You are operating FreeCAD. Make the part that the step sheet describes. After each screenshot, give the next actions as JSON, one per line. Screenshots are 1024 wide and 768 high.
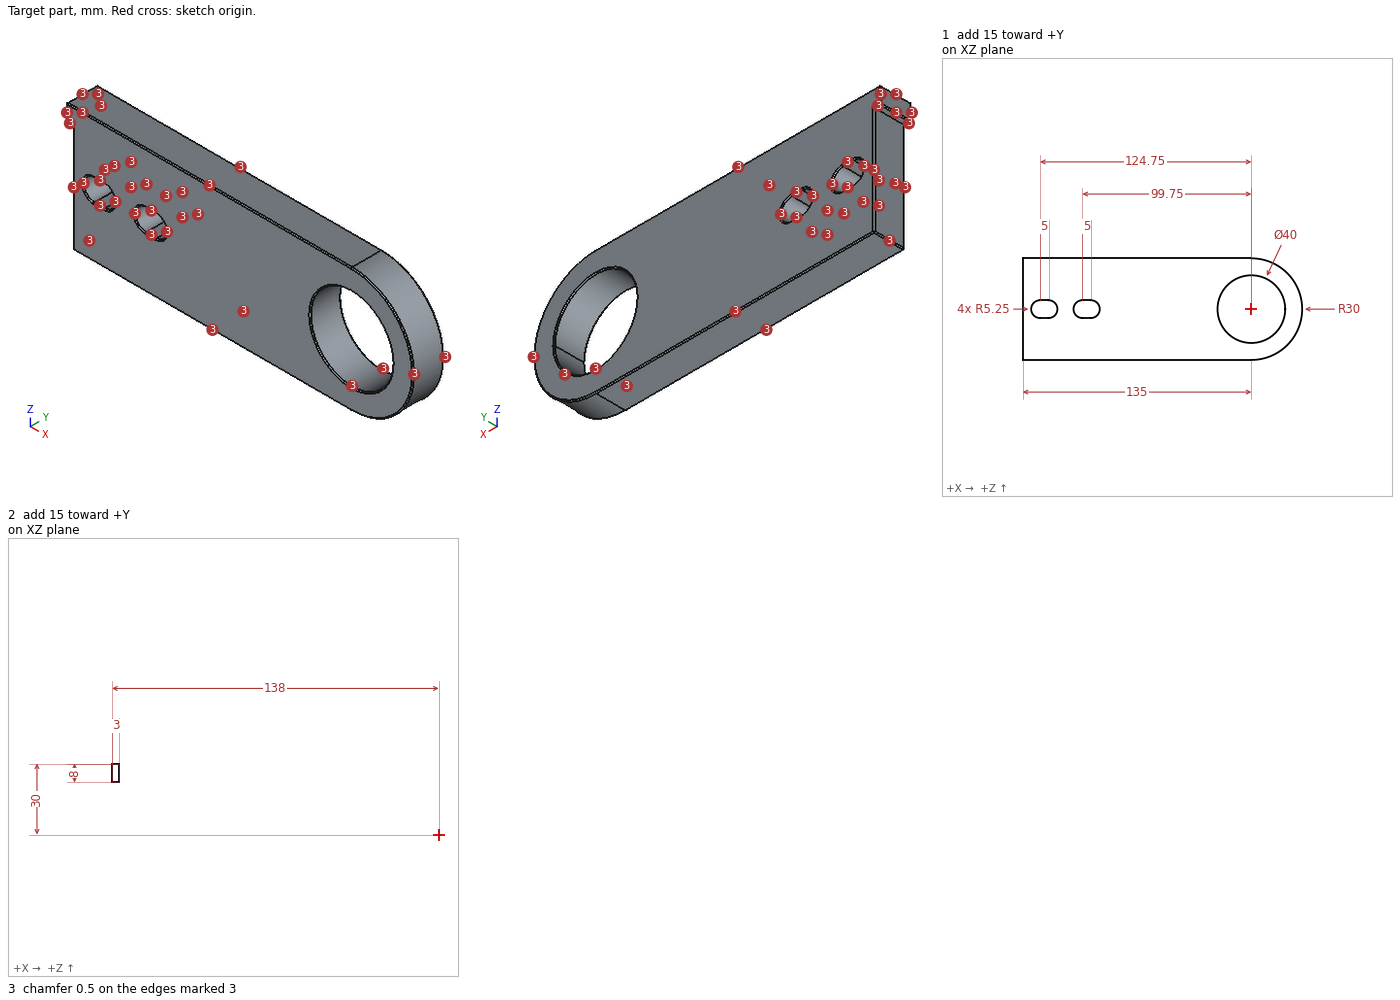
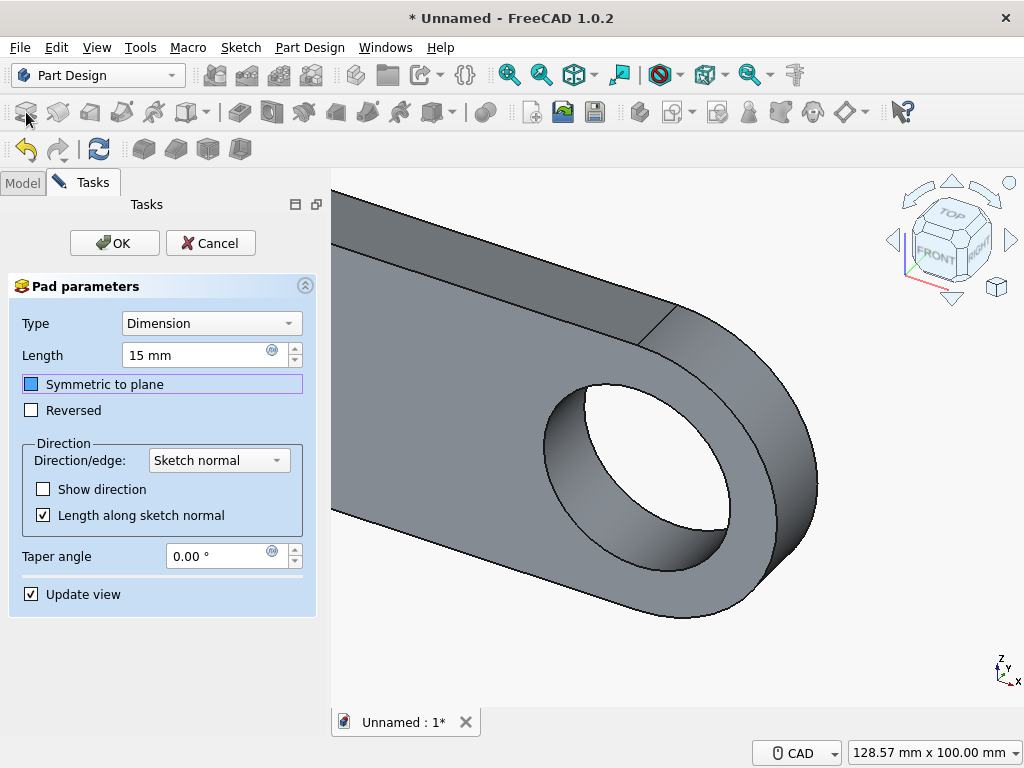
{"action": "left_click", "coordinate": [30, 410]}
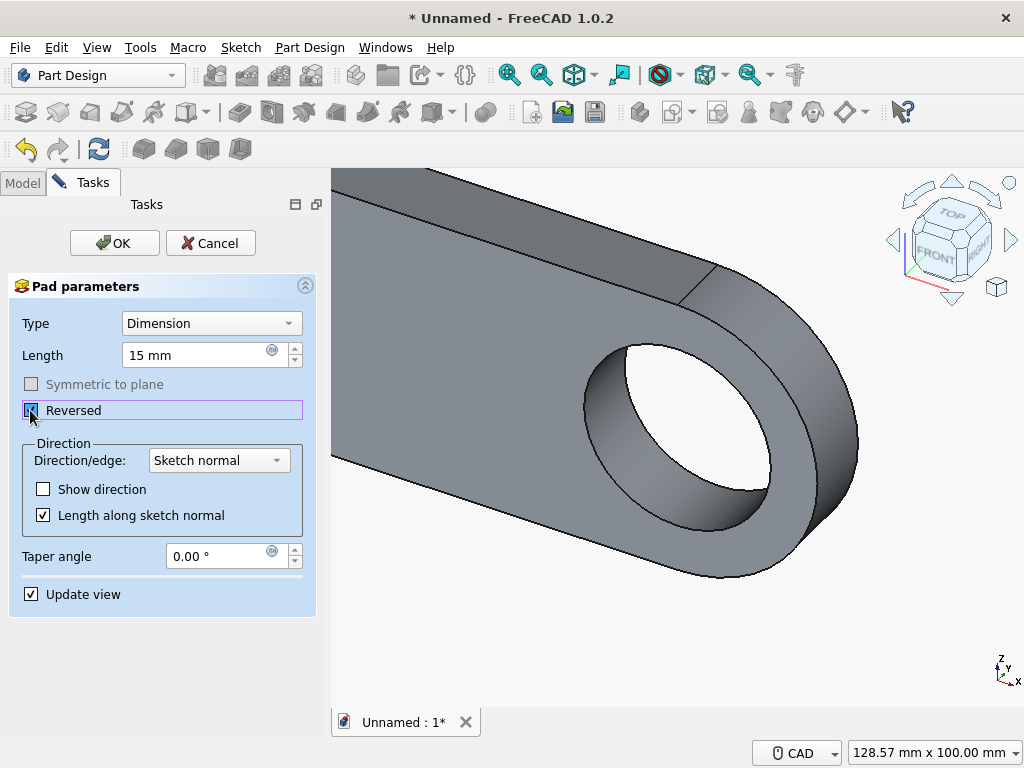
{"action": "left_click", "coordinate": [115, 243]}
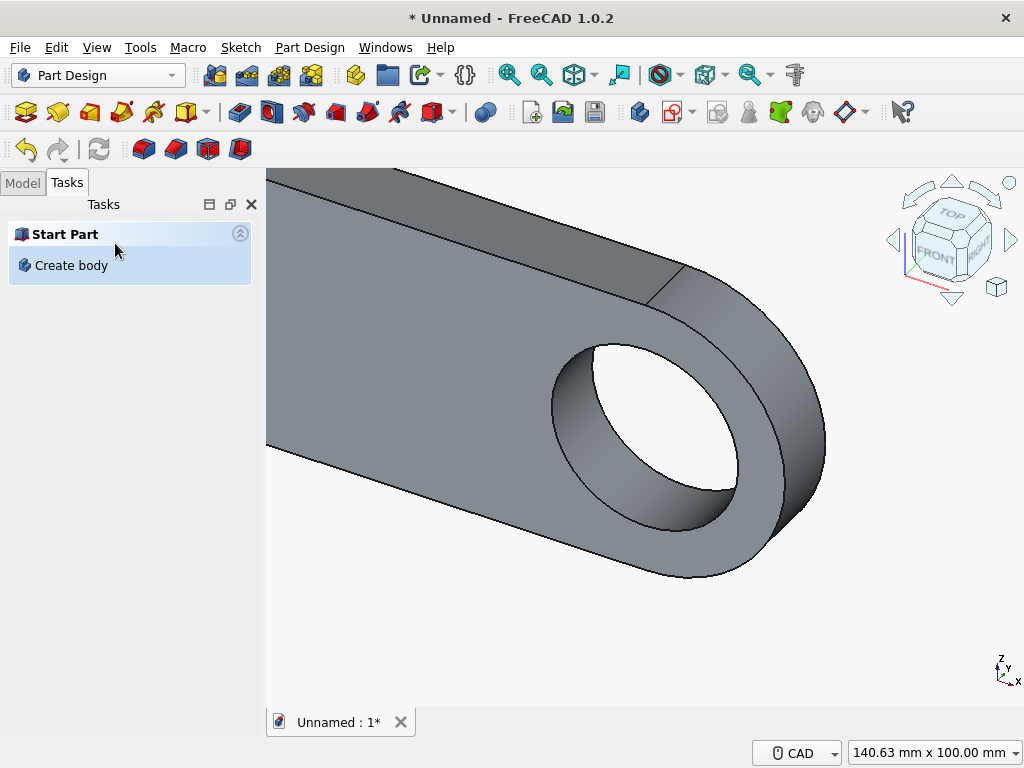
{"action": "left_click", "coordinate": [510, 76]}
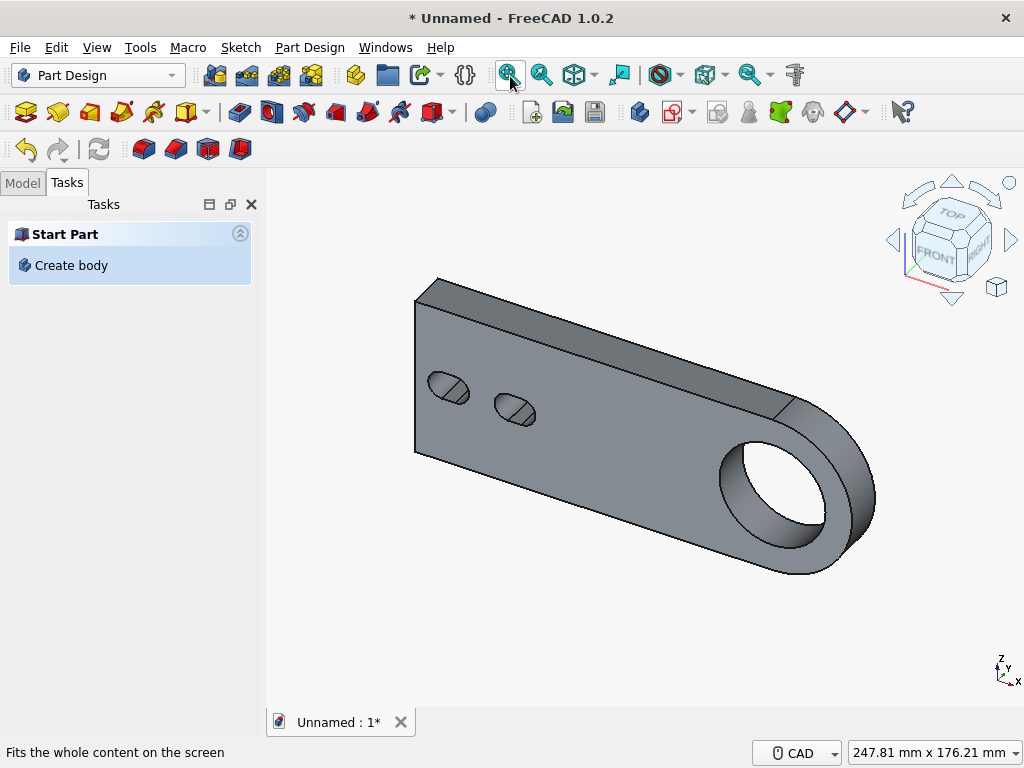
{"action": "left_click", "coordinate": [672, 112]}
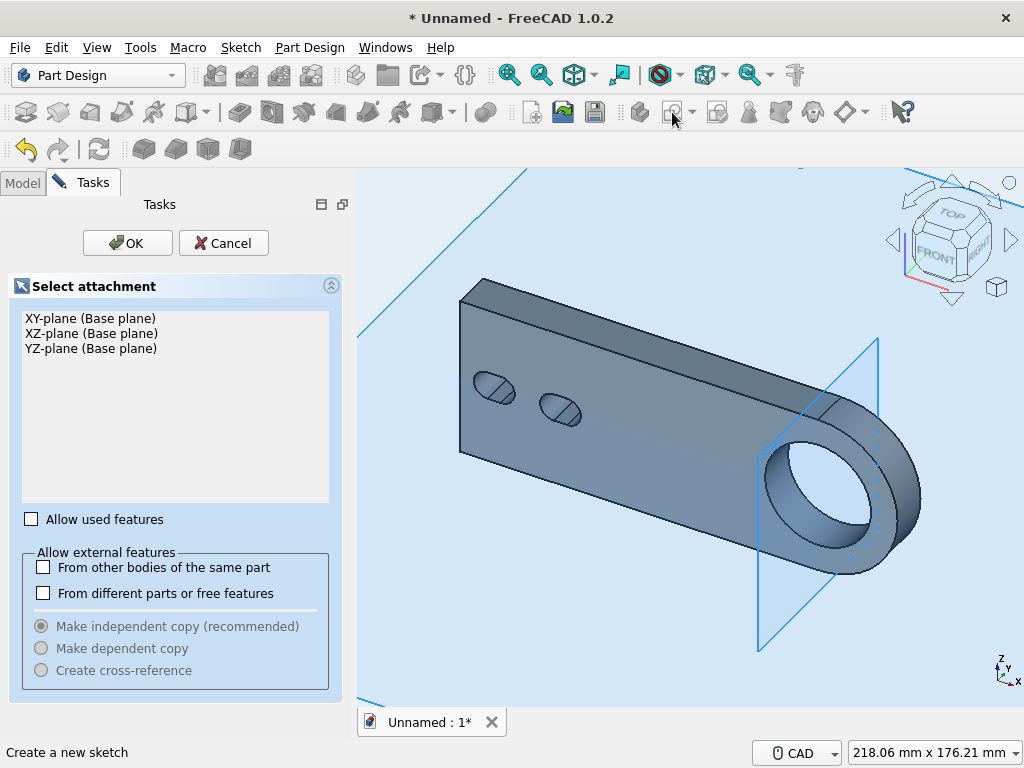
{"action": "left_click", "coordinate": [82, 334]}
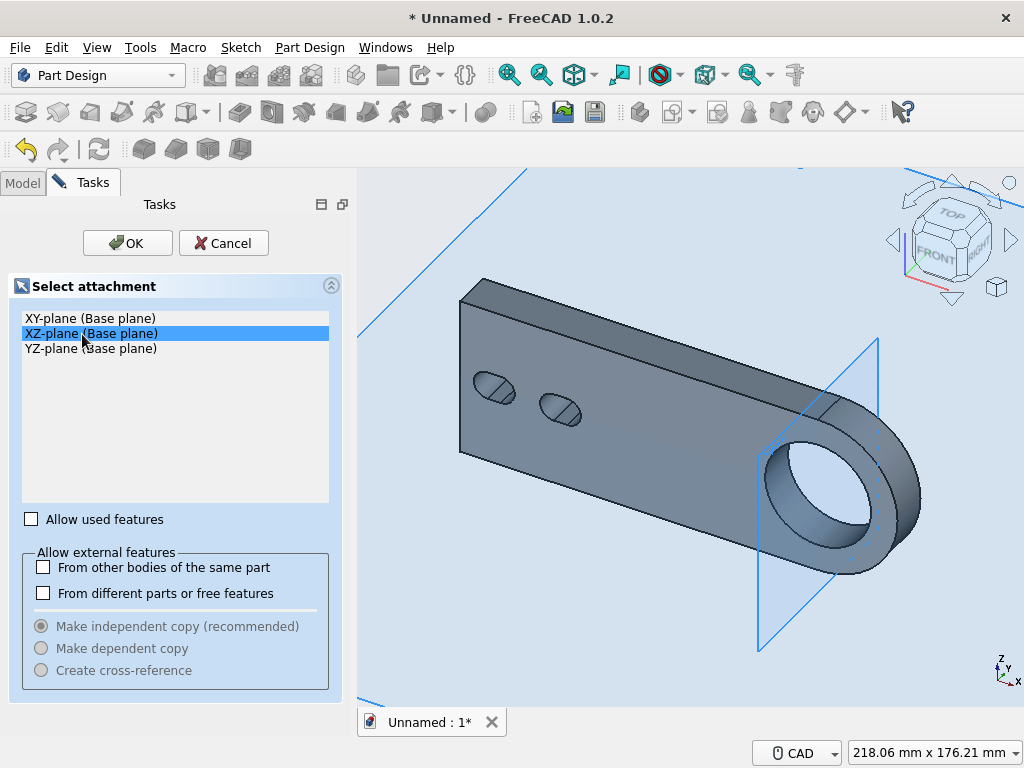
{"action": "left_click", "coordinate": [128, 243]}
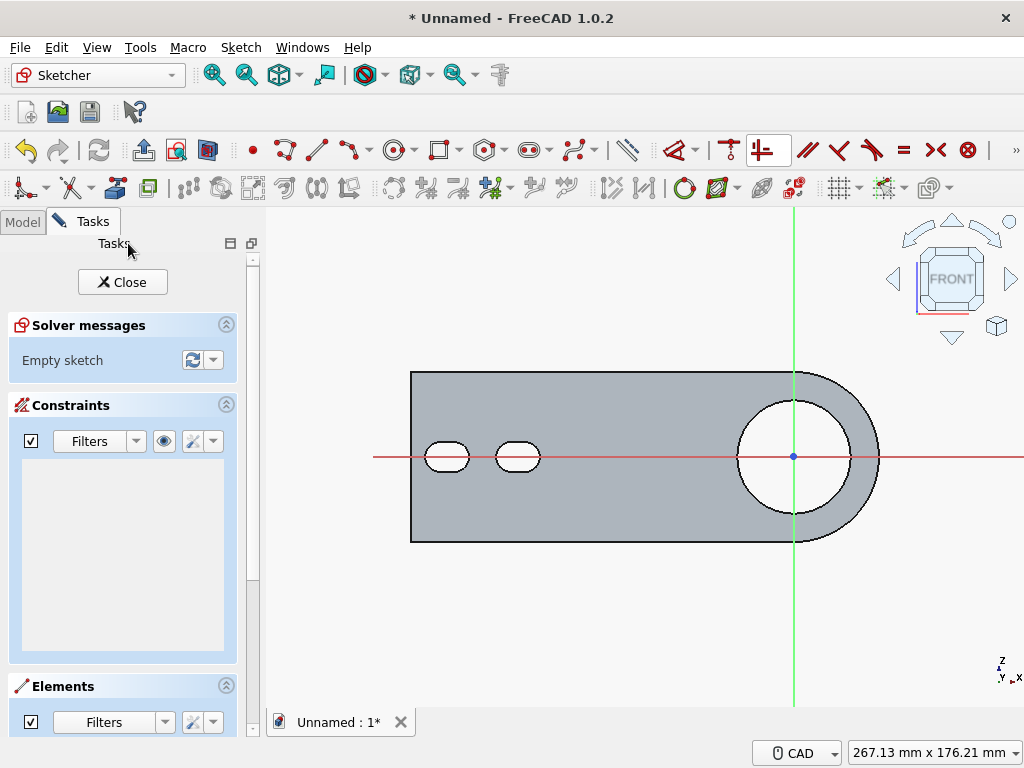
{"action": "scroll", "coordinate": [393, 377], "scroll_direction": "up", "scroll_amount": 13}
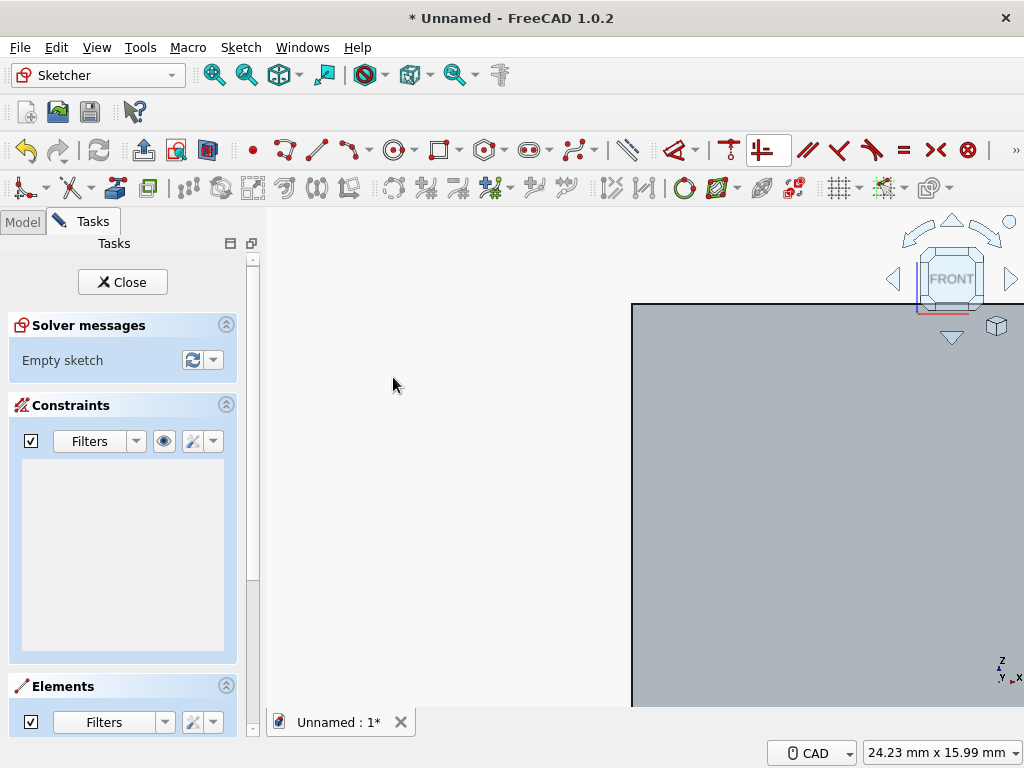
{"action": "left_click", "coordinate": [440, 150]}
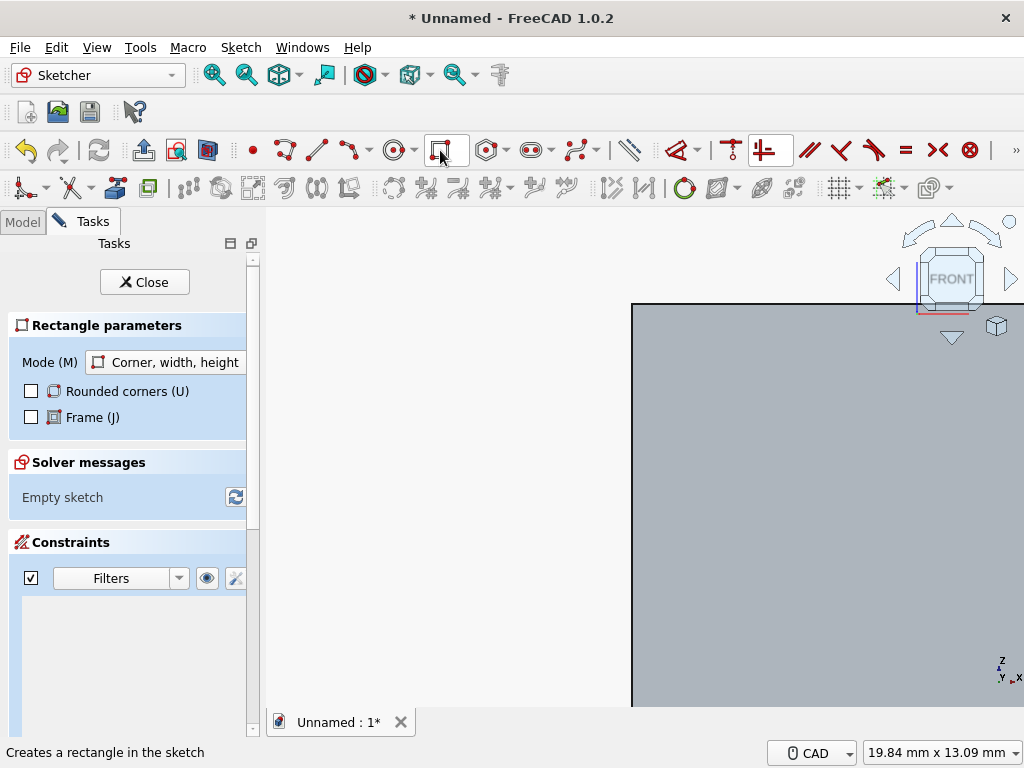
{"action": "left_click", "coordinate": [517, 304]}
{"action": "mouse_move", "coordinate": [632, 609]}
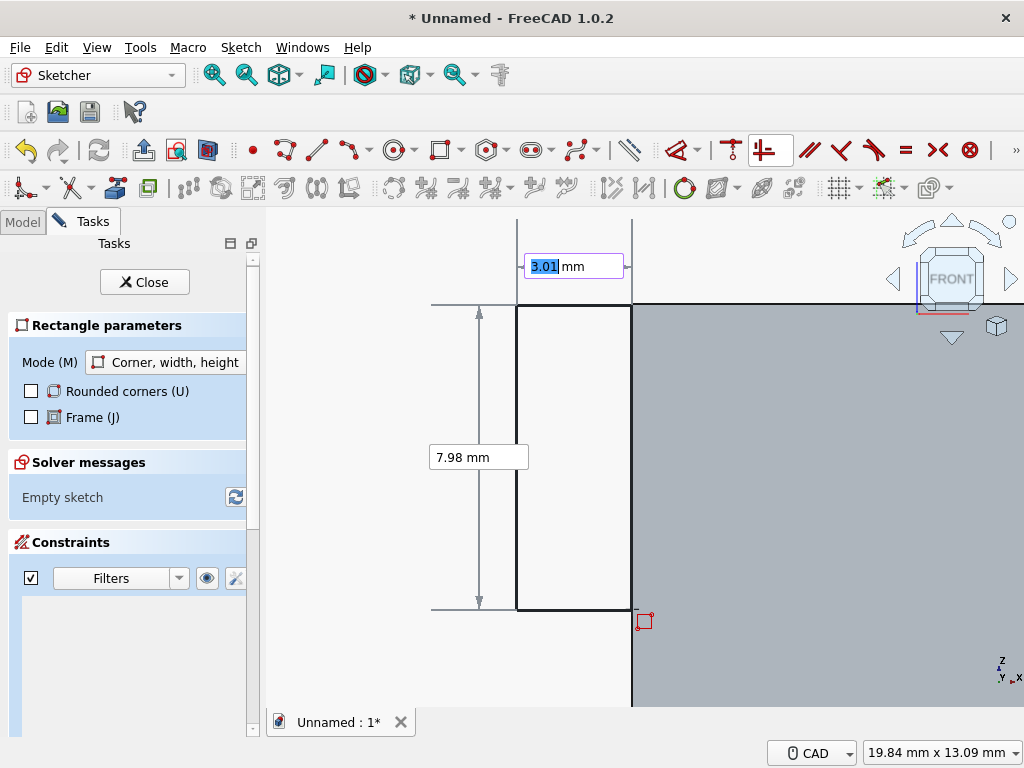
{"action": "type", "text": "3"}
{"action": "key", "text": "Tab"}
{"action": "type", "text": "8"}
{"action": "key", "text": "Return"}
{"action": "key", "text": "Escape"}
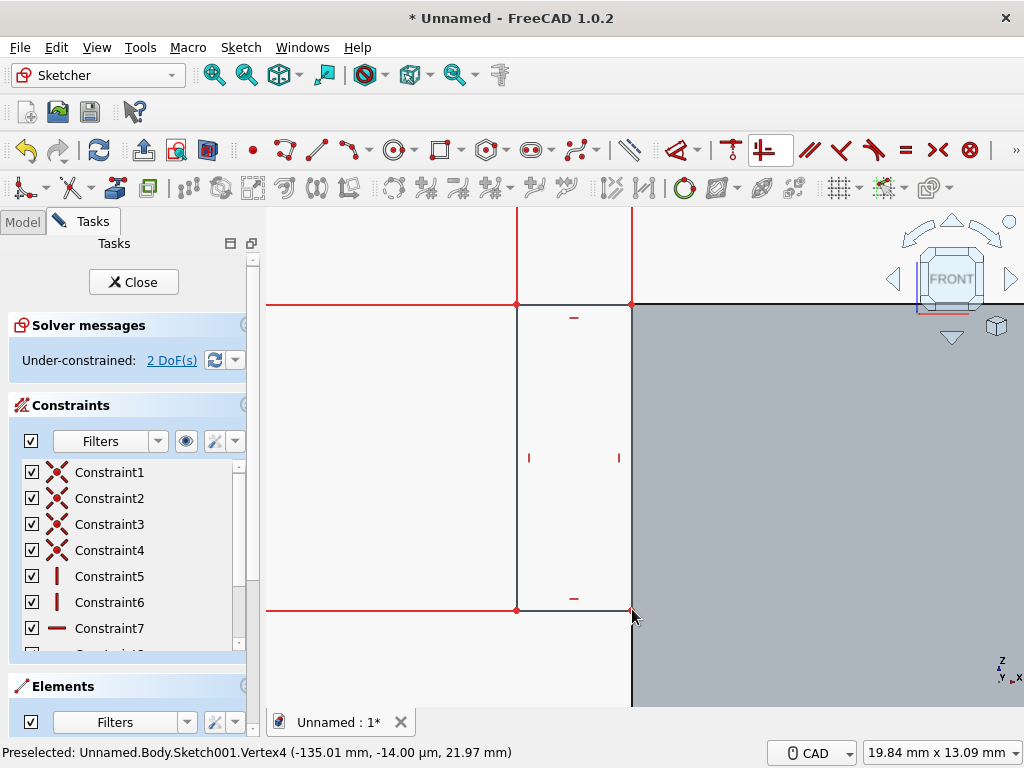
{"action": "left_click", "coordinate": [676, 150]}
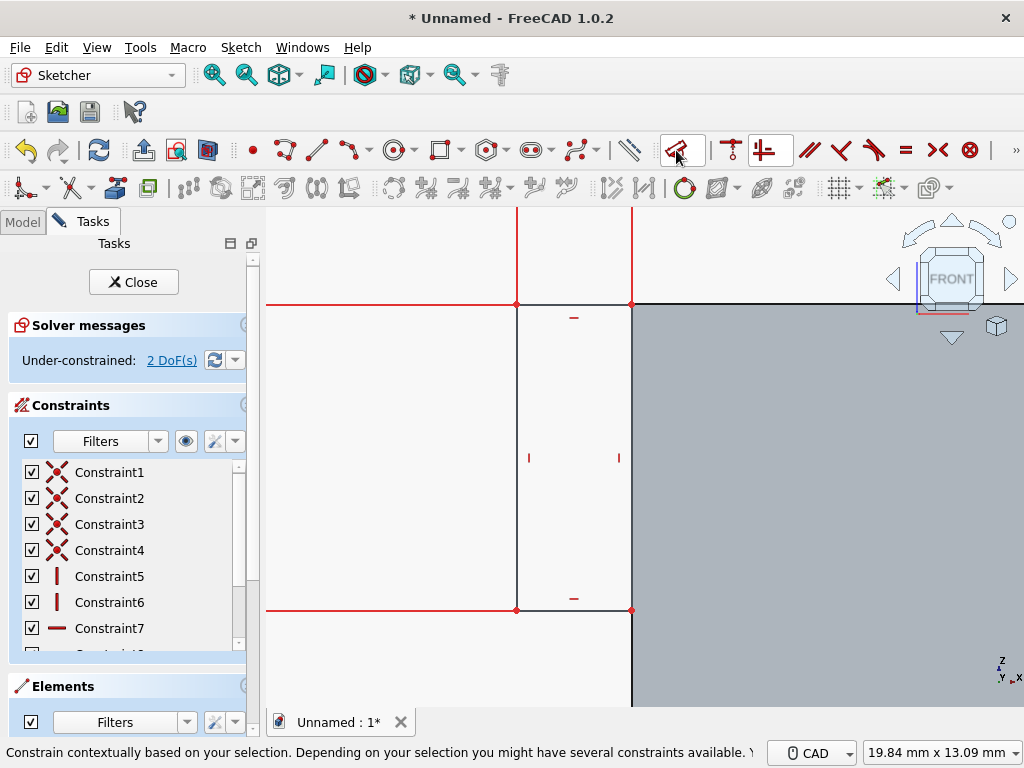
{"action": "left_click", "coordinate": [517, 305]}
{"action": "left_click", "coordinate": [483, 492]}